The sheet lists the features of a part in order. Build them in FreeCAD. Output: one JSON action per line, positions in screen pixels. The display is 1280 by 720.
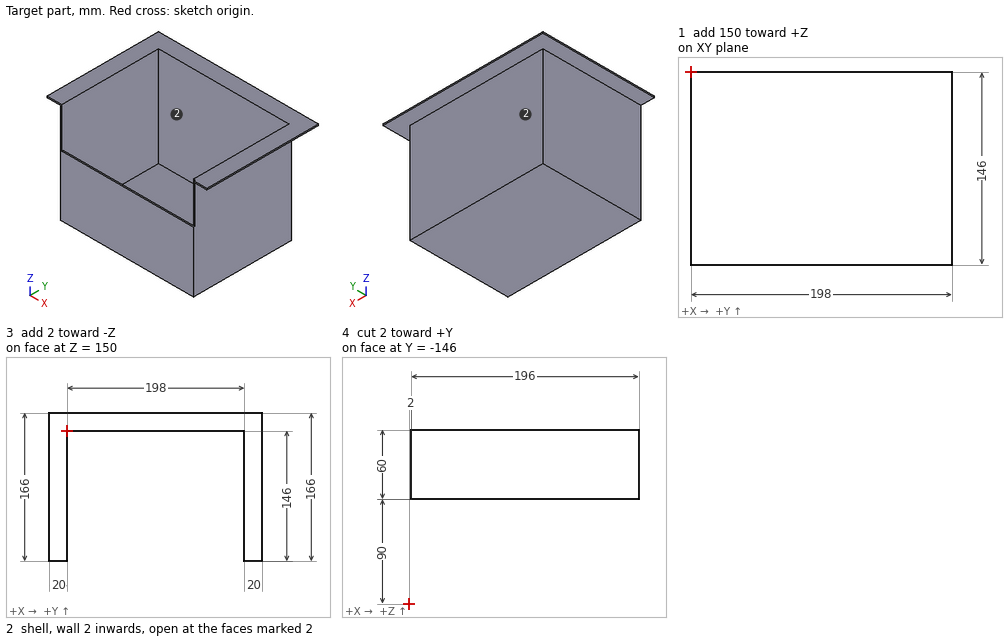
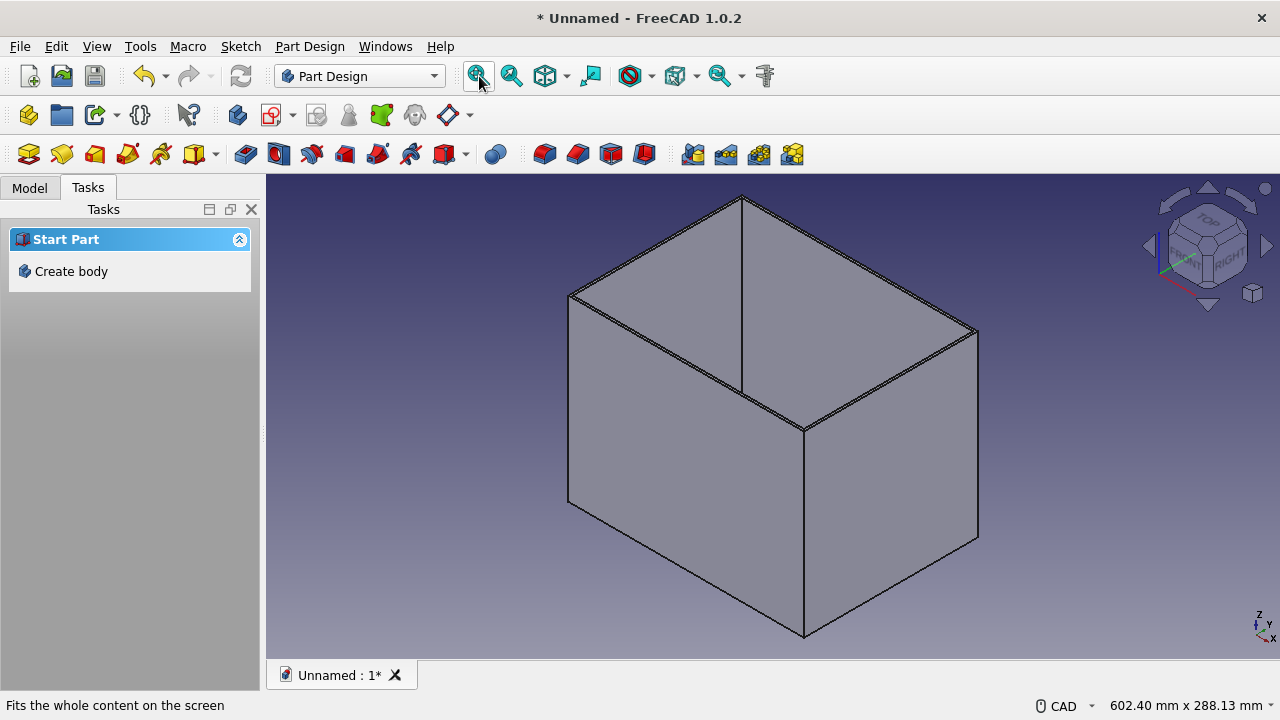
{"action": "scroll", "coordinate": [898, 286], "scroll_direction": "up", "scroll_amount": 12}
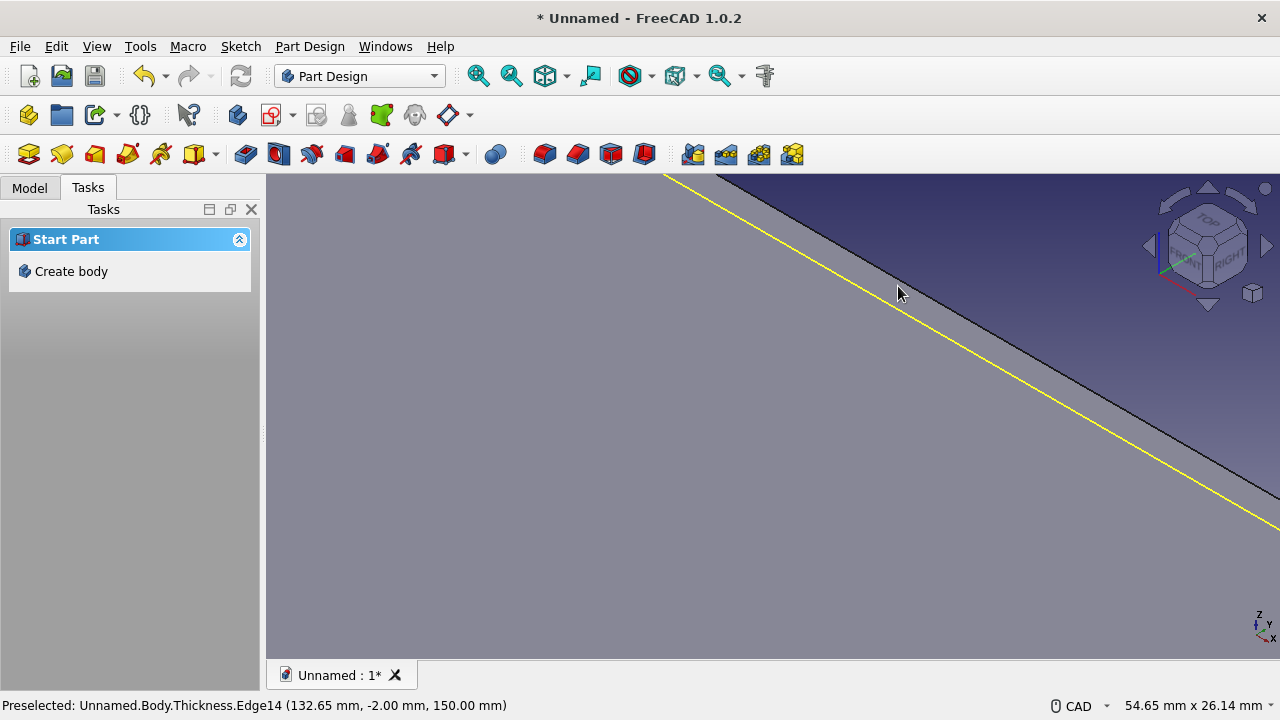
{"action": "left_click", "coordinate": [479, 76]}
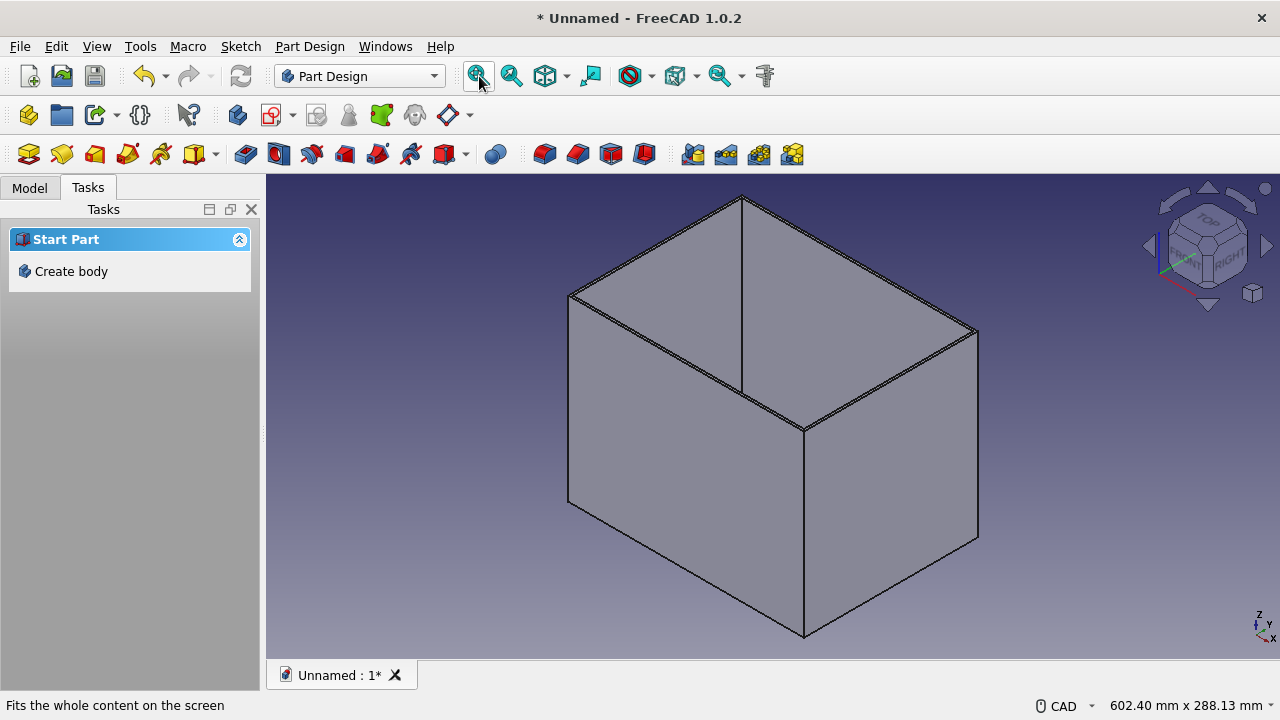
{"action": "key", "text": "2"}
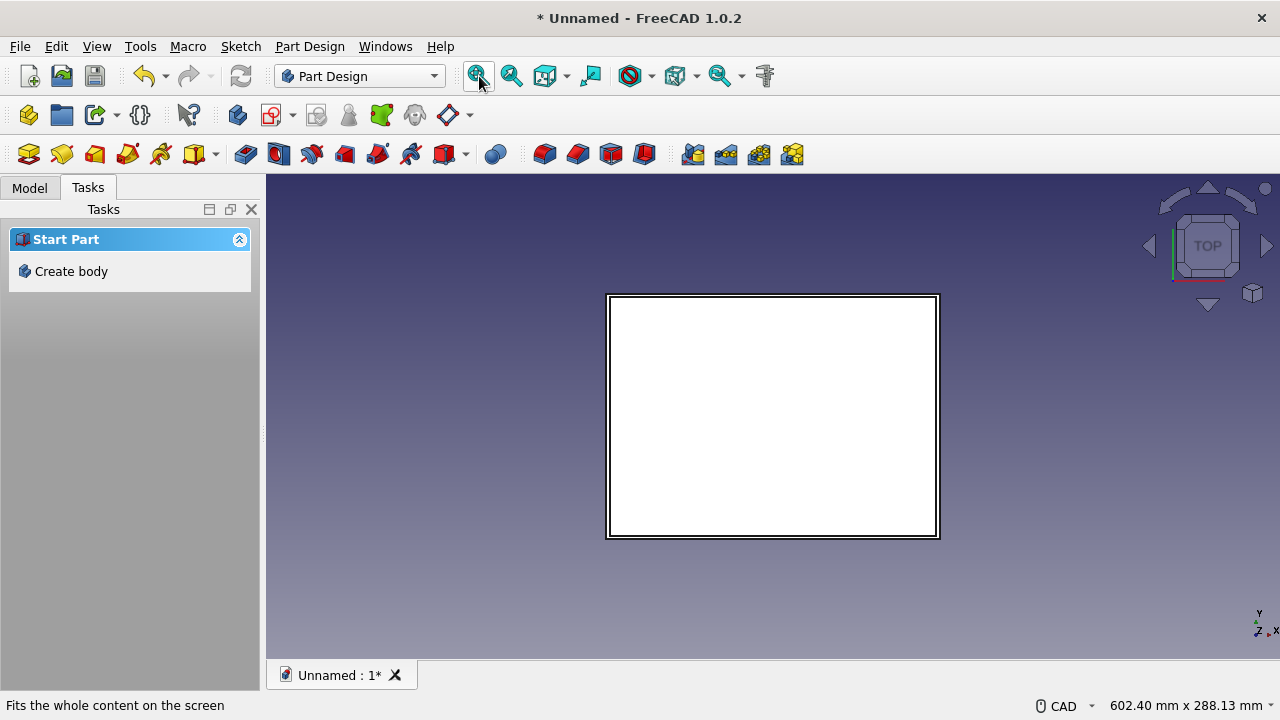
{"action": "scroll", "coordinate": [829, 295], "scroll_direction": "up", "scroll_amount": 12}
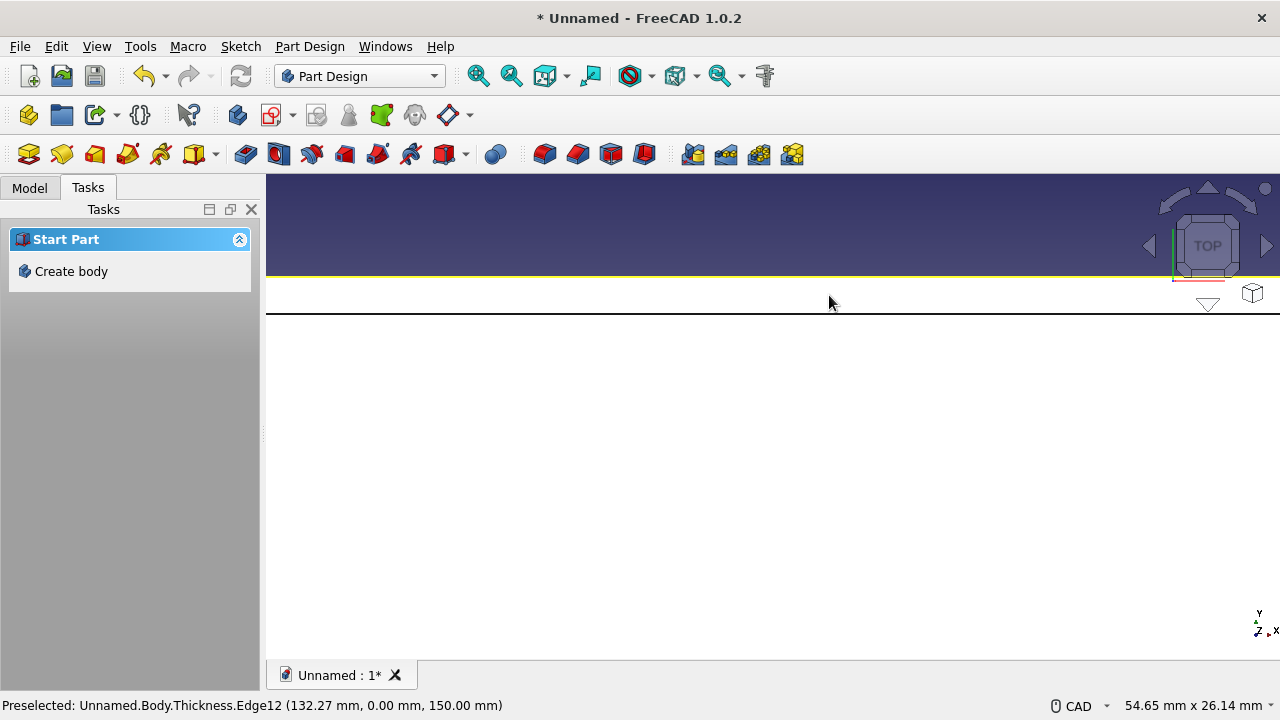
{"action": "left_click", "coordinate": [818, 301]}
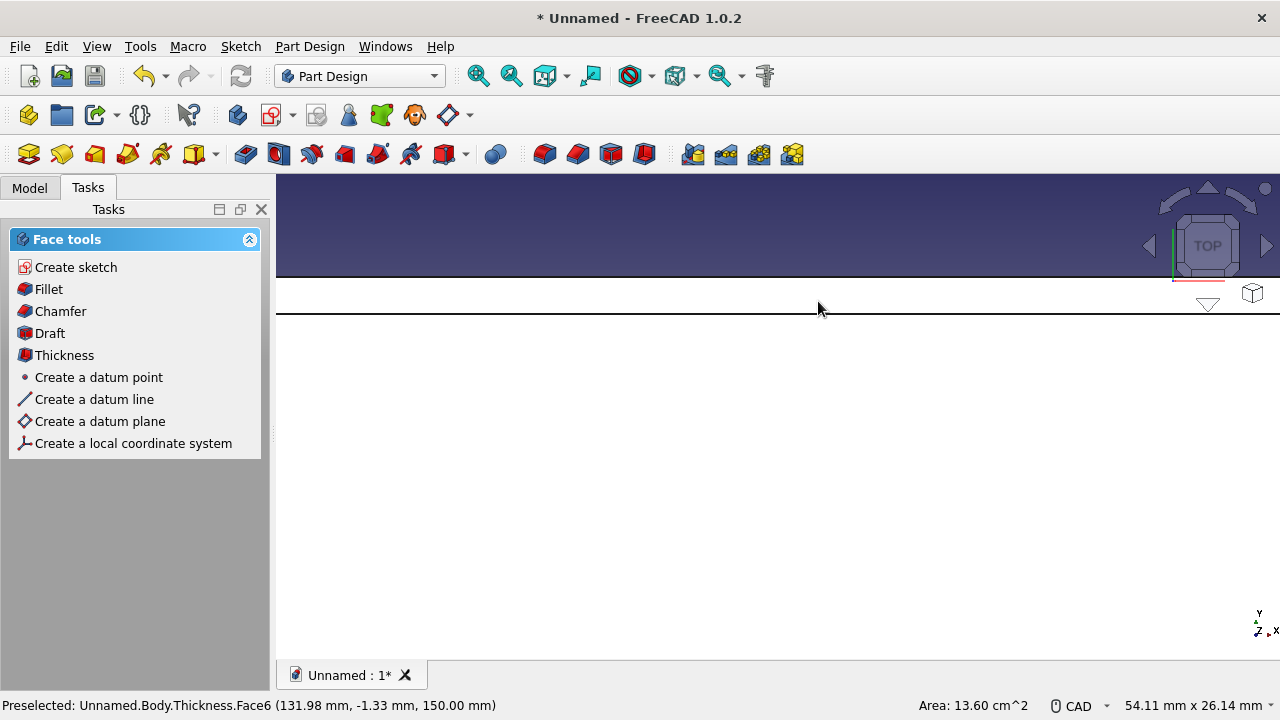
{"action": "left_click", "coordinate": [270, 116]}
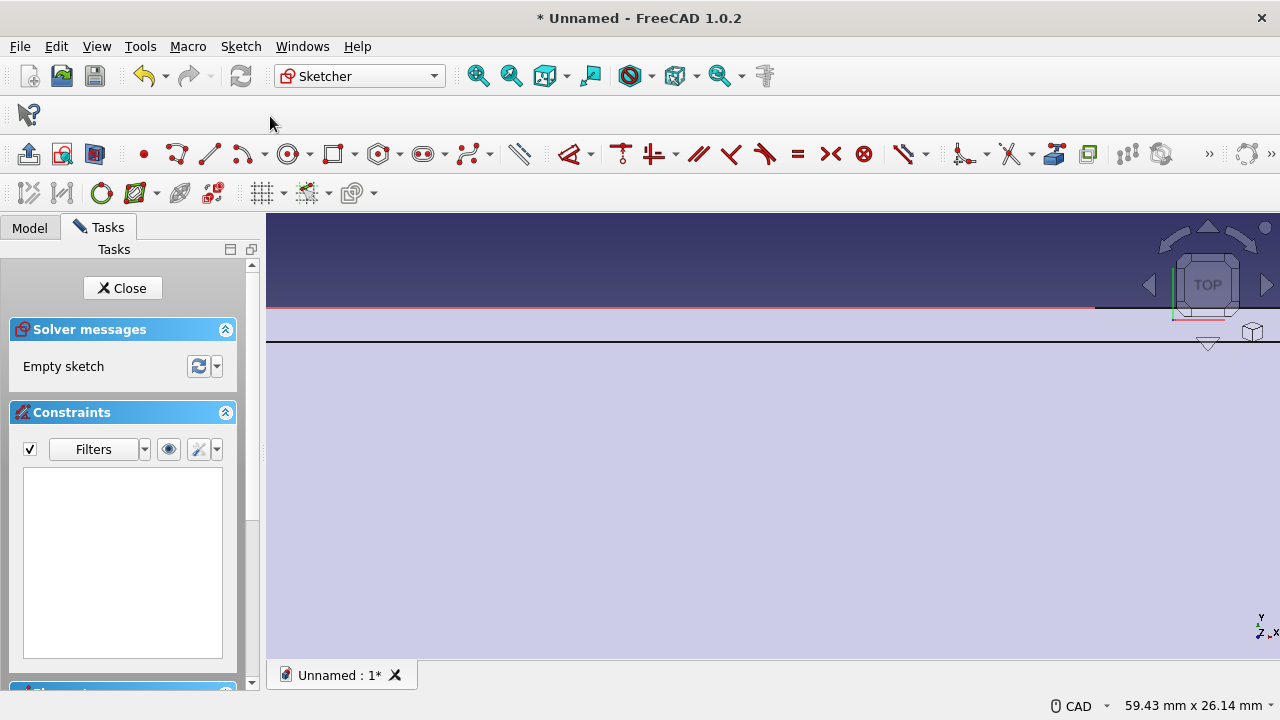
{"action": "scroll", "coordinate": [750, 342], "scroll_direction": "down", "scroll_amount": 12}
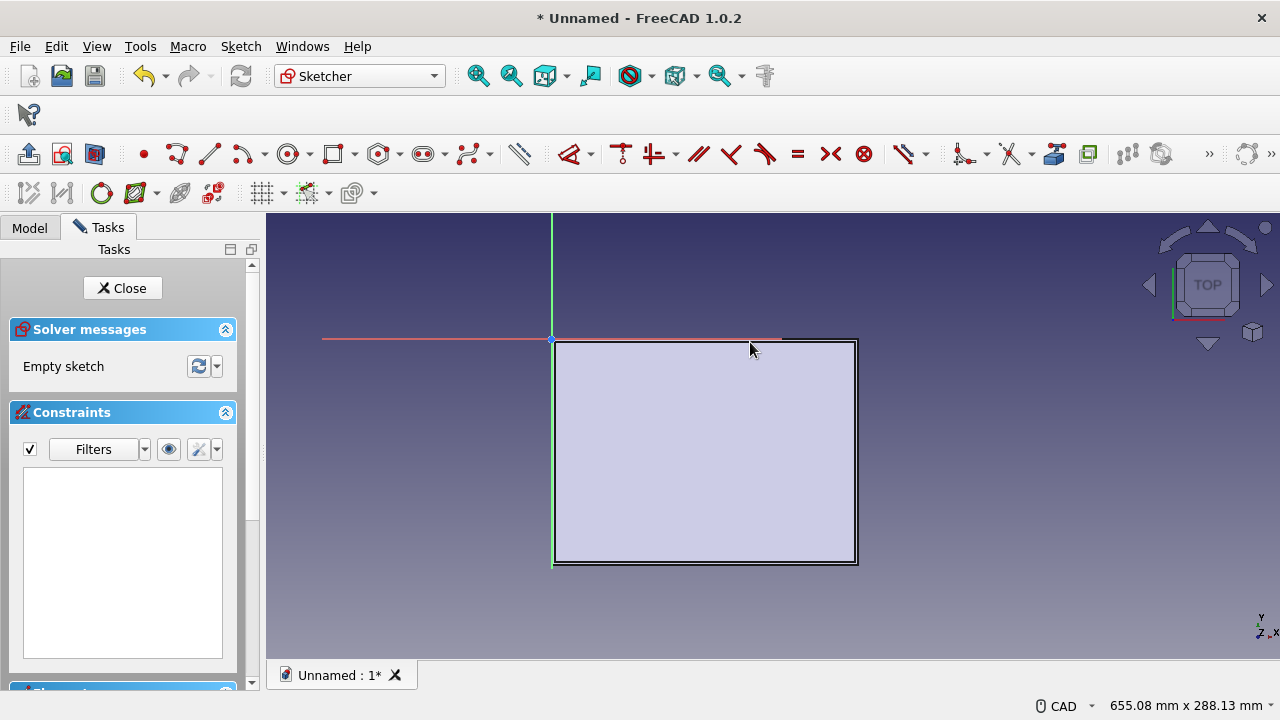
{"action": "left_click", "coordinate": [177, 154]}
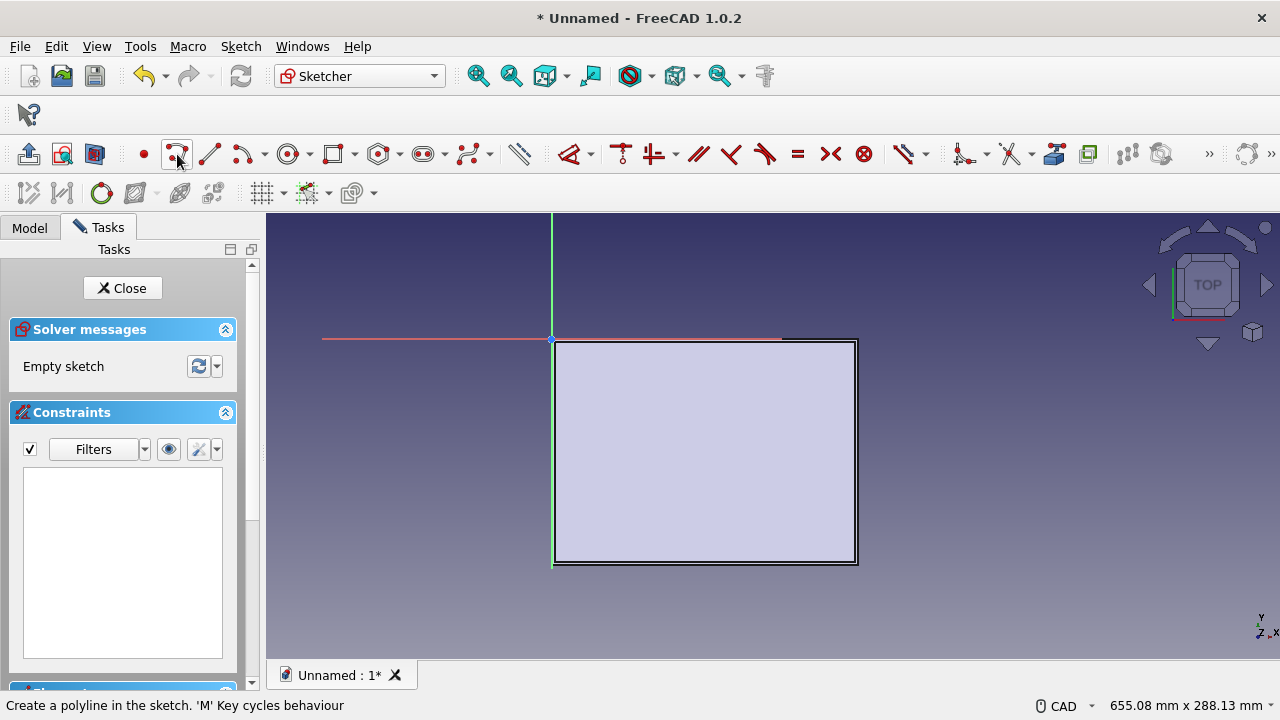
{"action": "left_click", "coordinate": [552, 339]}
{"action": "left_click", "coordinate": [858, 348]}
{"action": "left_click", "coordinate": [858, 565]}
{"action": "left_click", "coordinate": [889, 565]}
{"action": "left_click", "coordinate": [889, 308]}
{"action": "left_click", "coordinate": [521, 308]}
{"action": "left_click", "coordinate": [521, 565]}
{"action": "left_click", "coordinate": [561, 565]}
{"action": "left_click", "coordinate": [552, 339]}
{"action": "key", "text": "Escape"}
{"action": "key", "text": "Escape"}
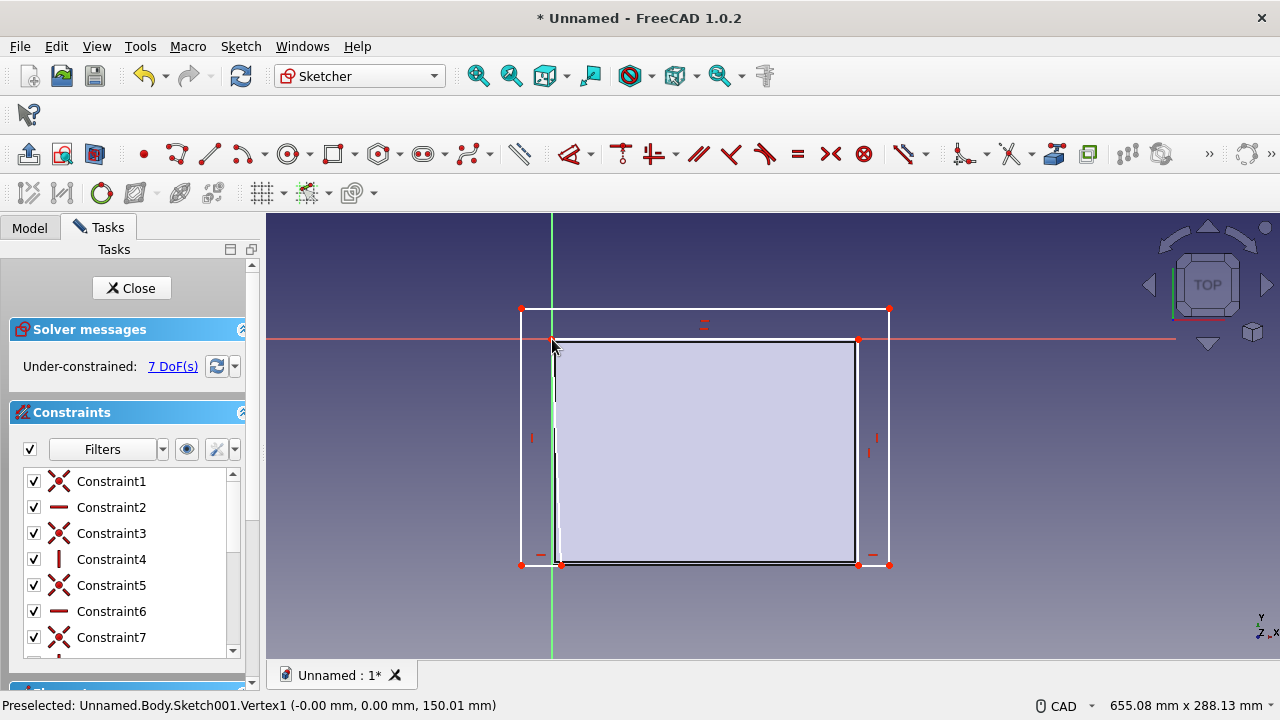
{"action": "left_click", "coordinate": [555, 407]}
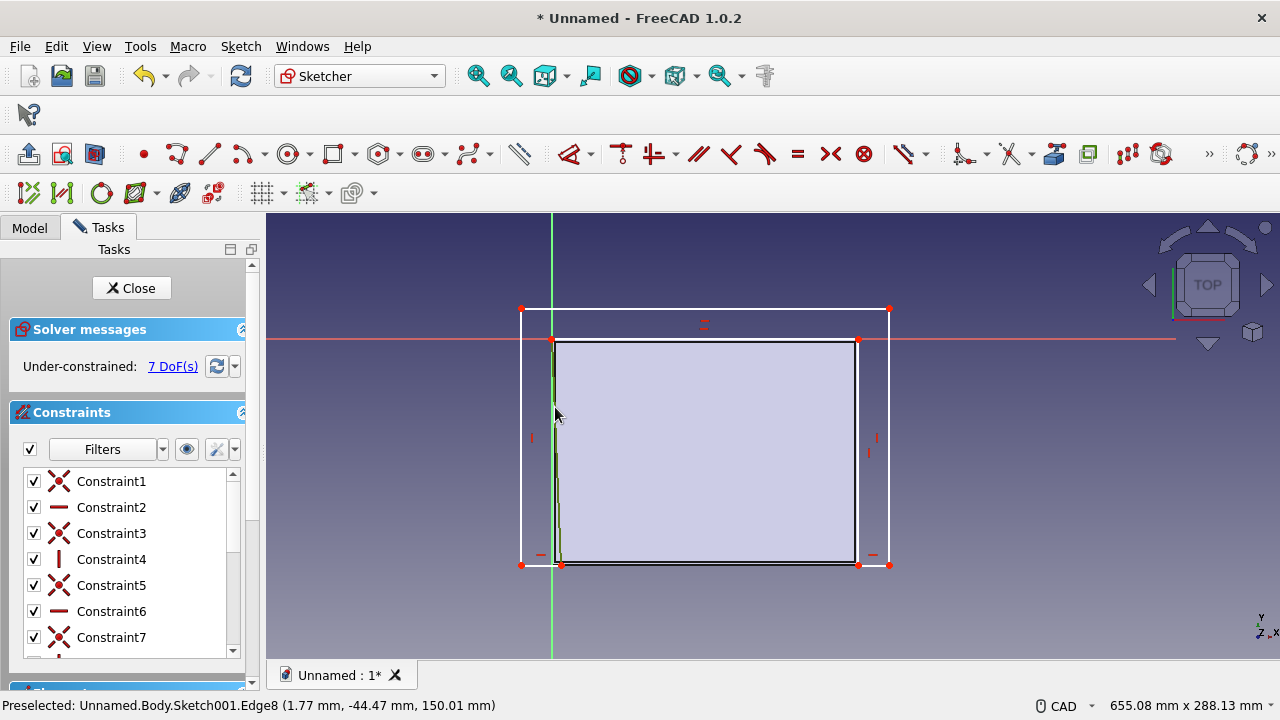
{"action": "left_click", "coordinate": [676, 154]}